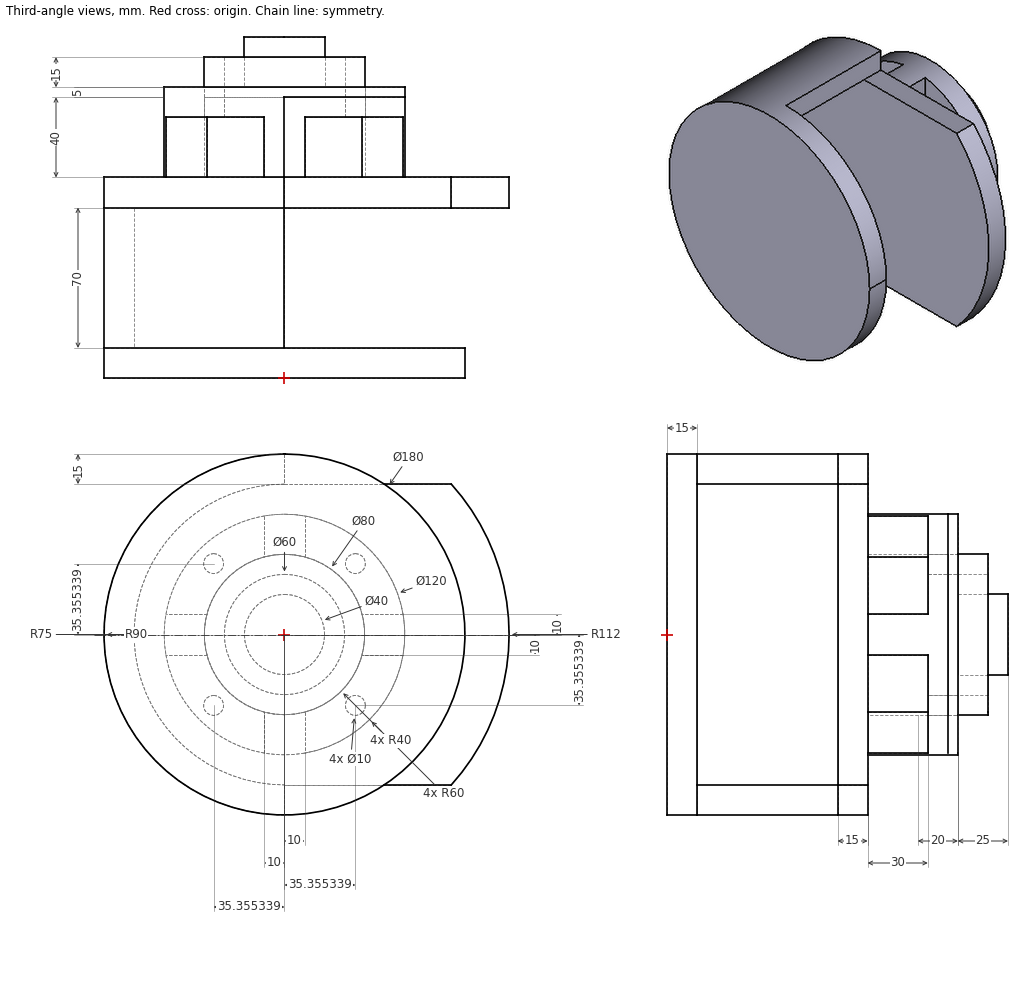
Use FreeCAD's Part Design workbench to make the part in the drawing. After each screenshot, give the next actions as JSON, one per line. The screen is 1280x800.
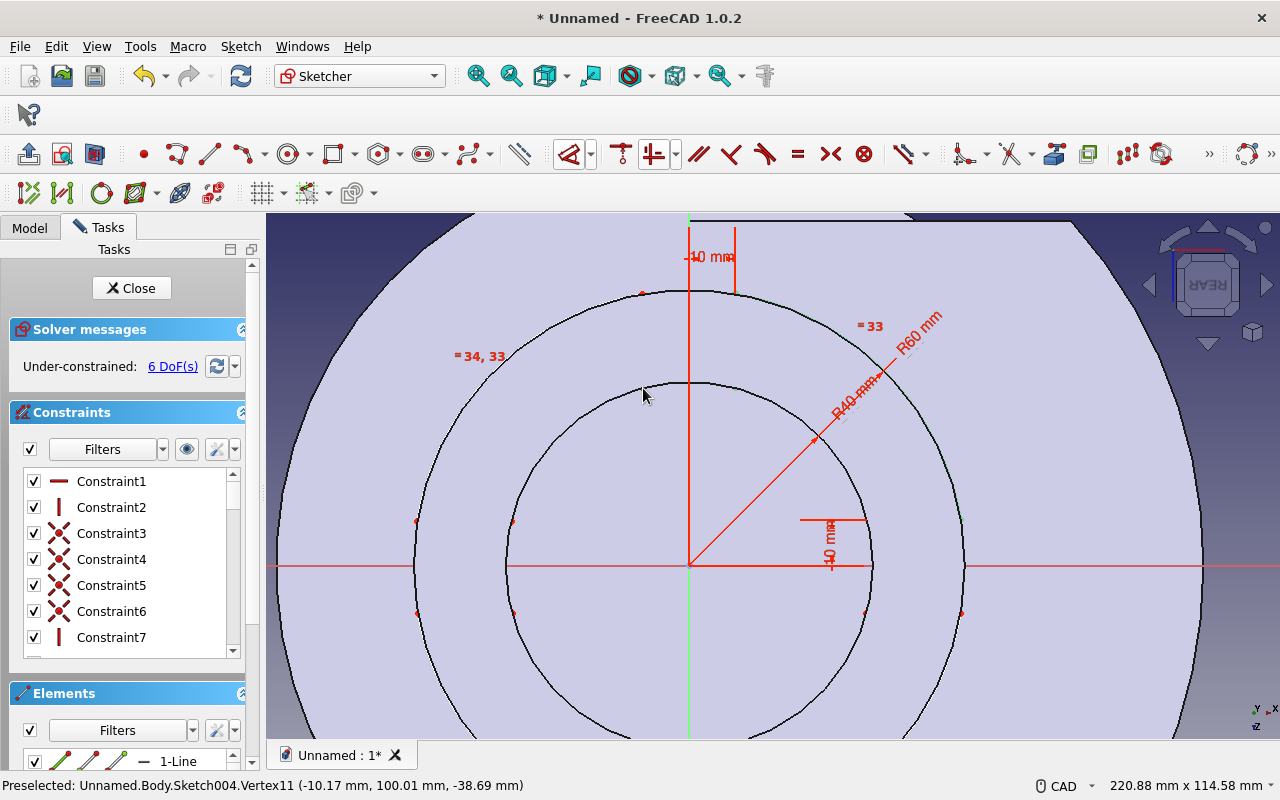
{"action": "key", "text": "l"}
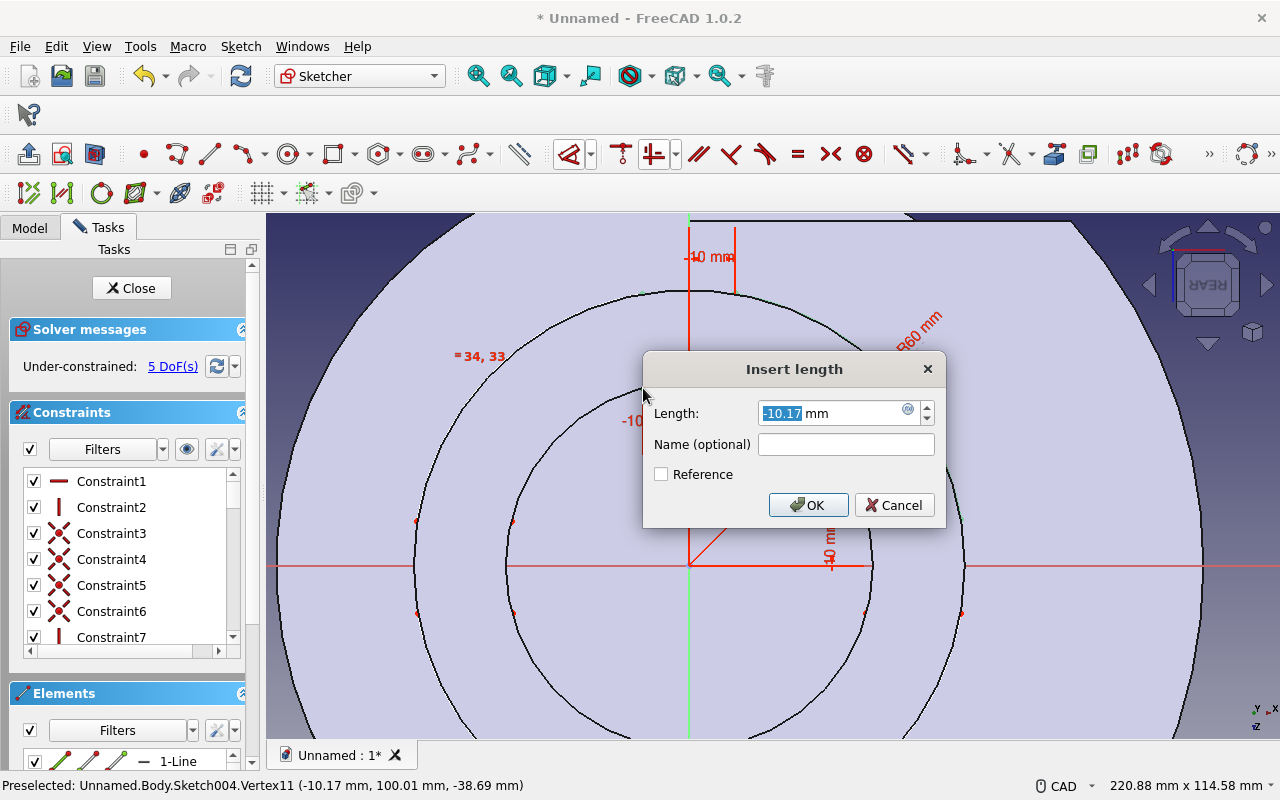
{"action": "type", "text": "-10"}
{"action": "key", "text": "Return"}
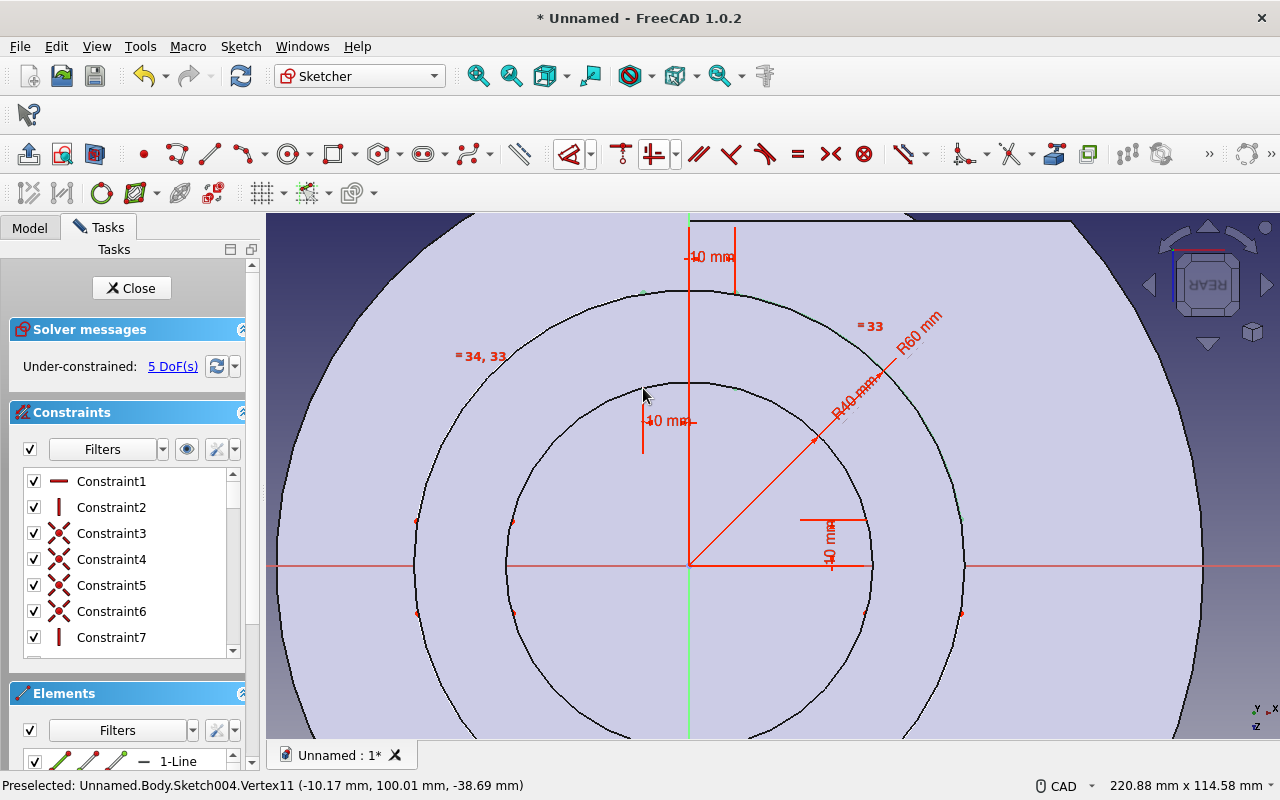
{"action": "left_click", "coordinate": [417, 521]}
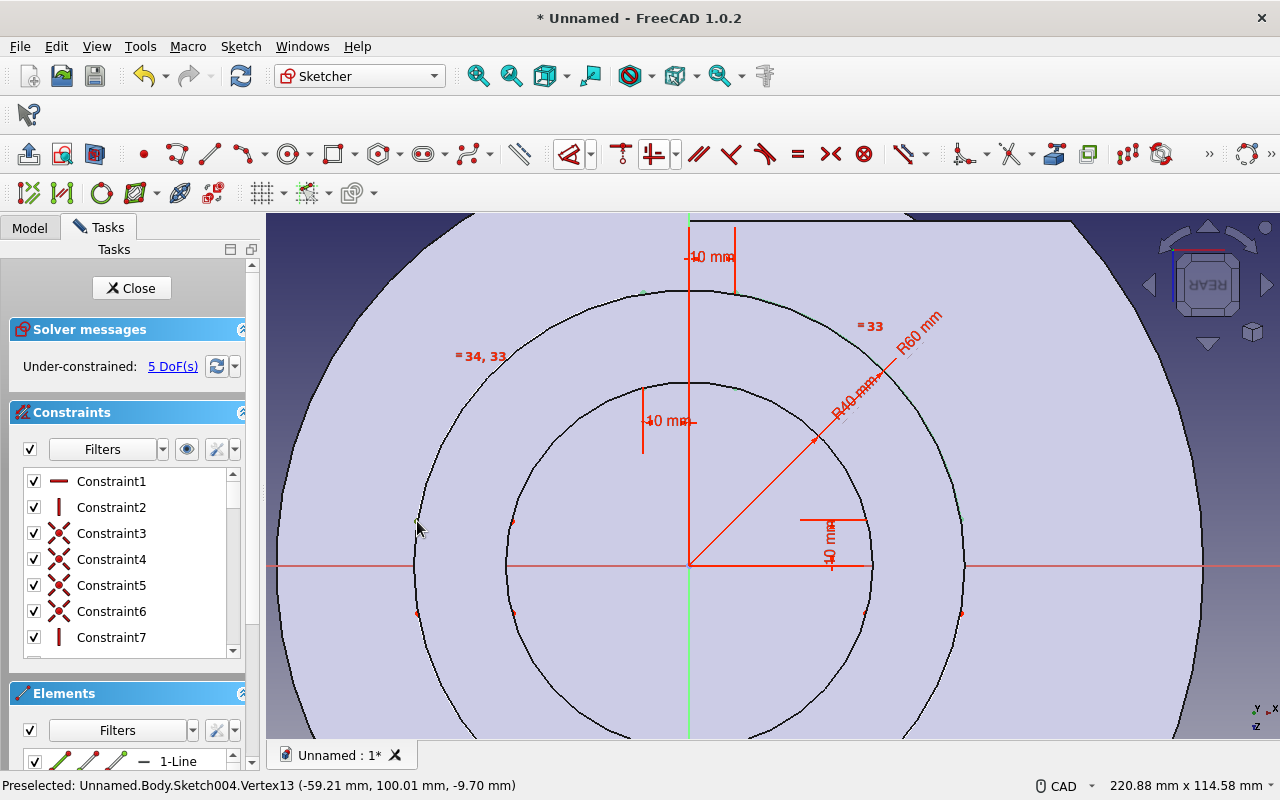
{"action": "key", "text": "i"}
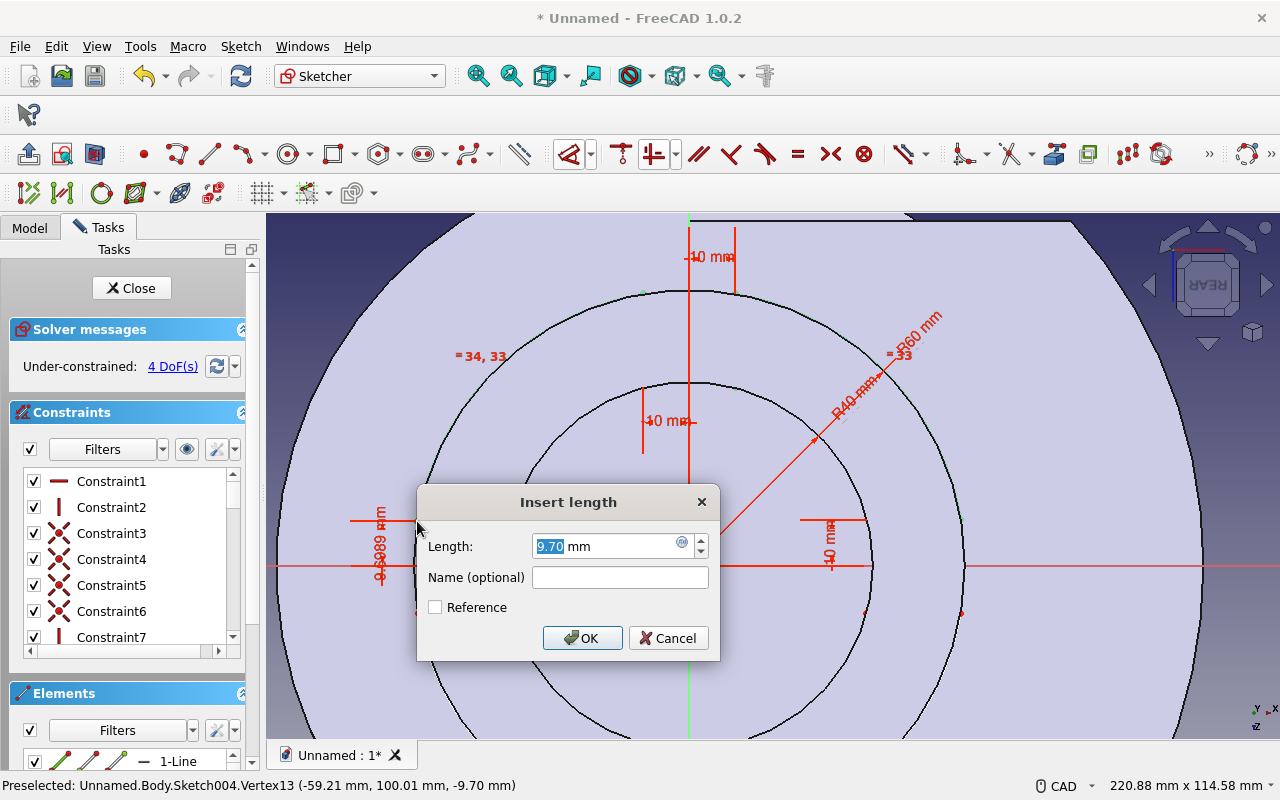
{"action": "type", "text": "10"}
{"action": "key", "text": "Return"}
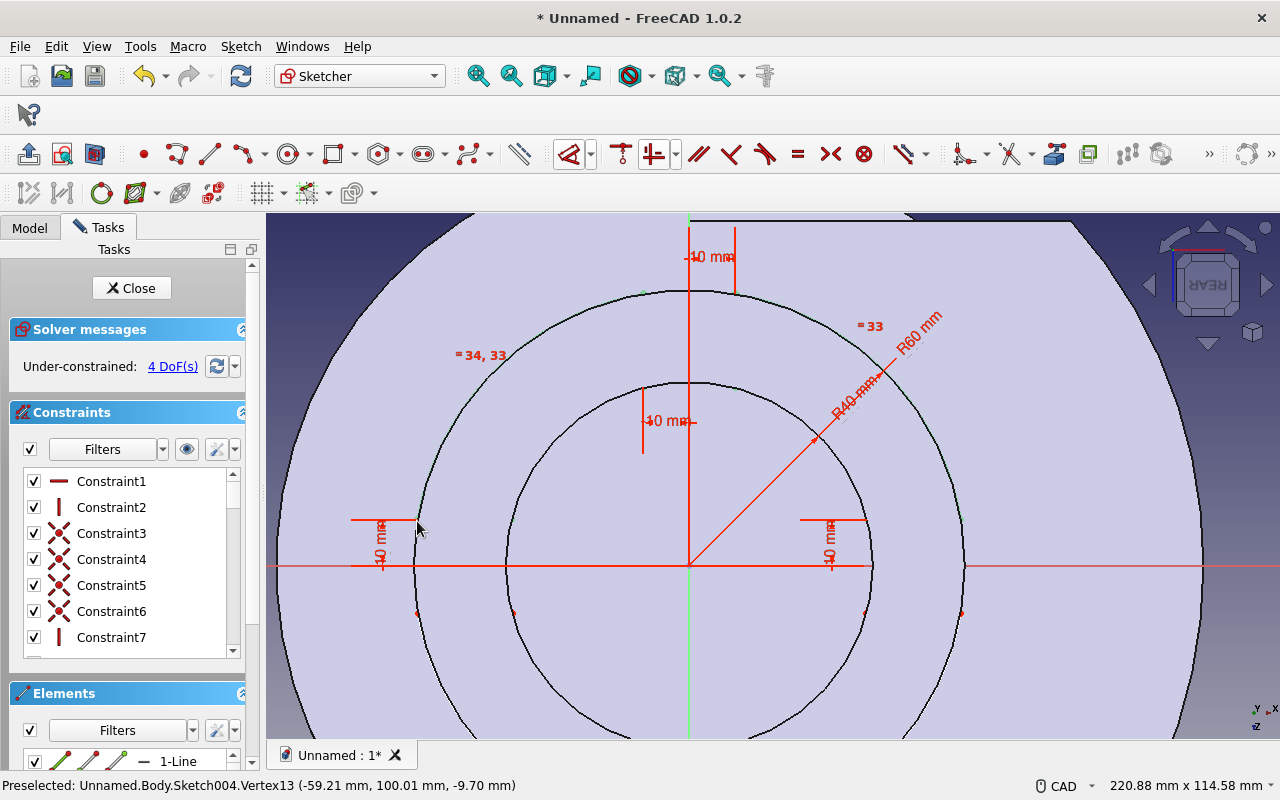
{"action": "left_click", "coordinate": [960, 614]}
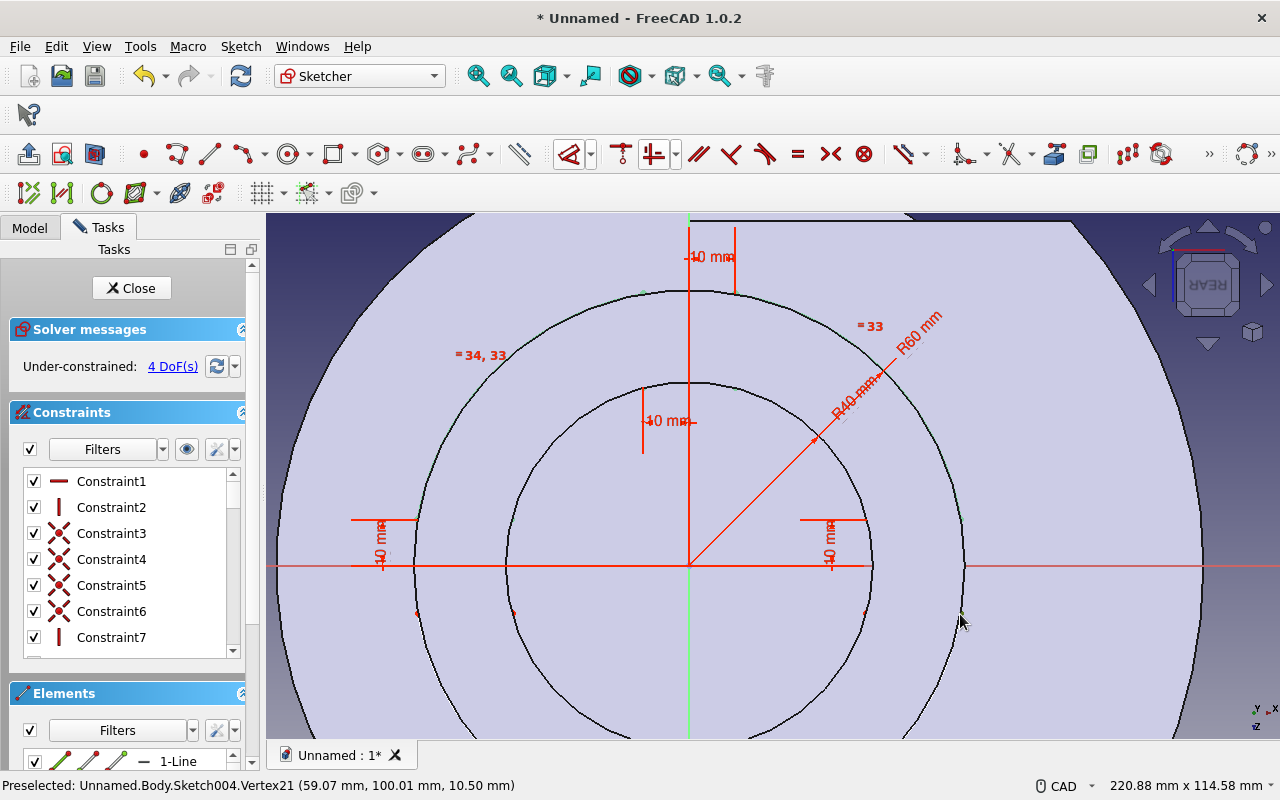
{"action": "key", "text": "i"}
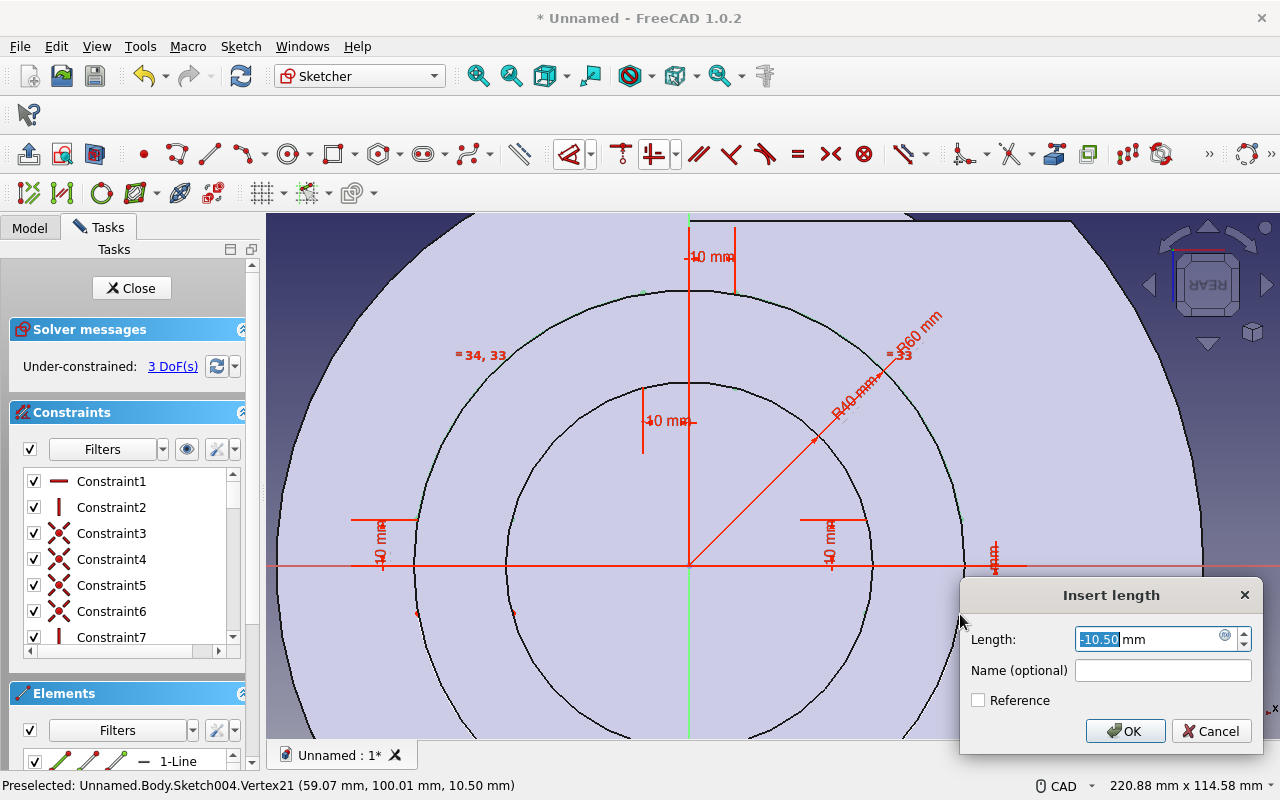
{"action": "type", "text": "-10"}
{"action": "key", "text": "Return"}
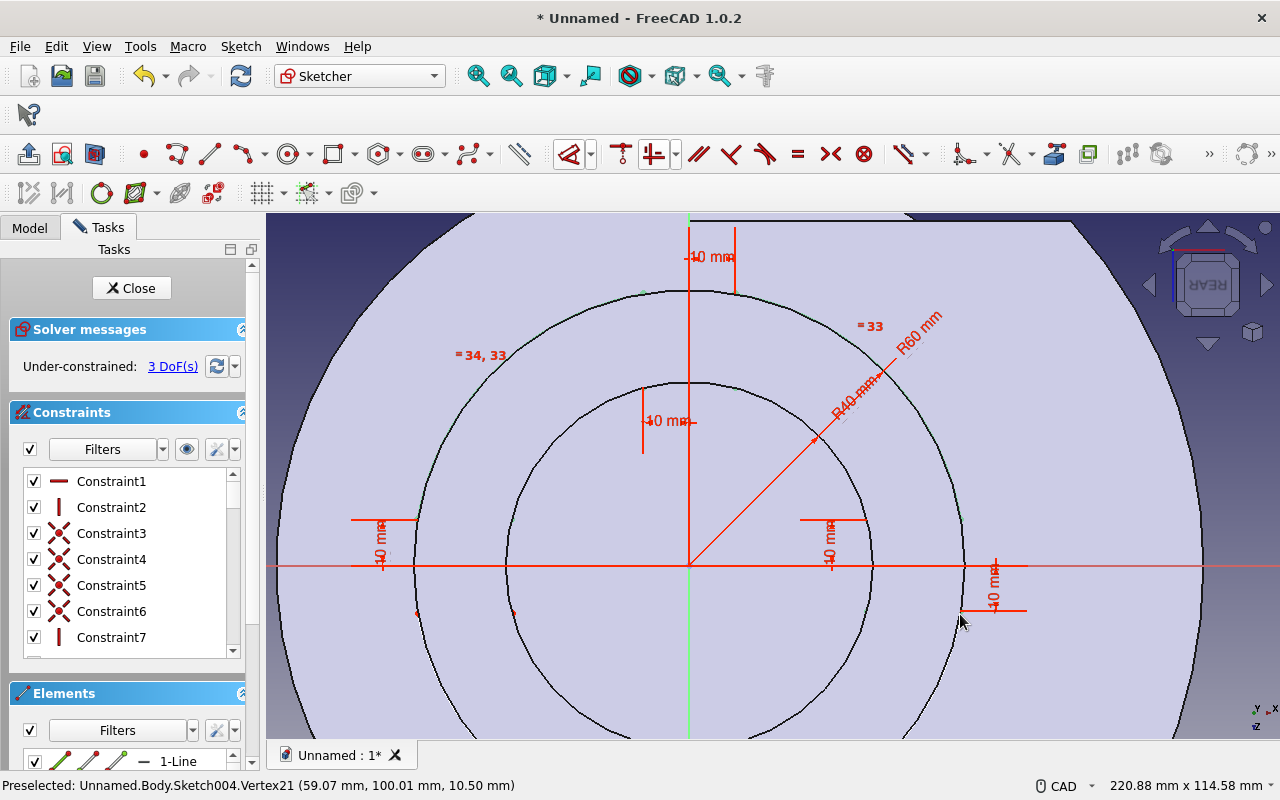
{"action": "scroll", "coordinate": [735, 294], "scroll_direction": "down", "scroll_amount": 2}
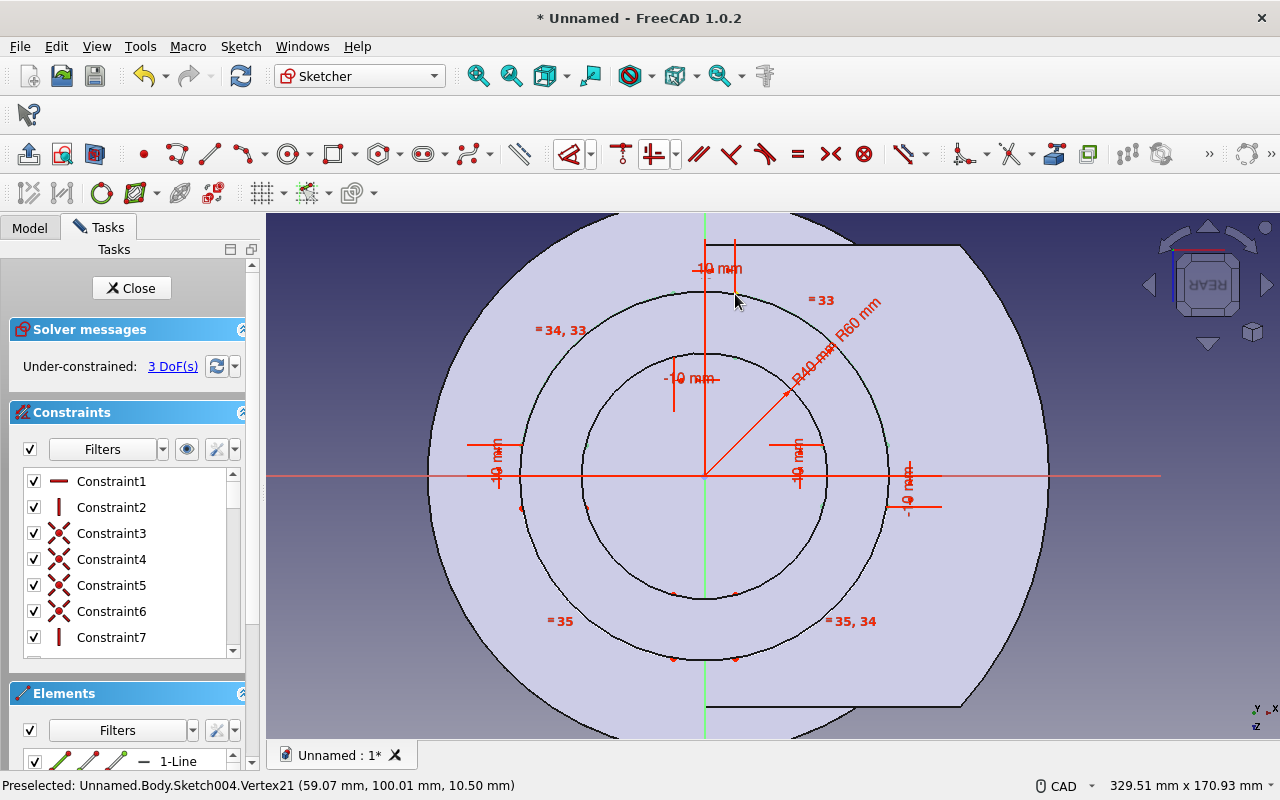
{"action": "scroll", "coordinate": [735, 595], "scroll_direction": "up", "scroll_amount": 2}